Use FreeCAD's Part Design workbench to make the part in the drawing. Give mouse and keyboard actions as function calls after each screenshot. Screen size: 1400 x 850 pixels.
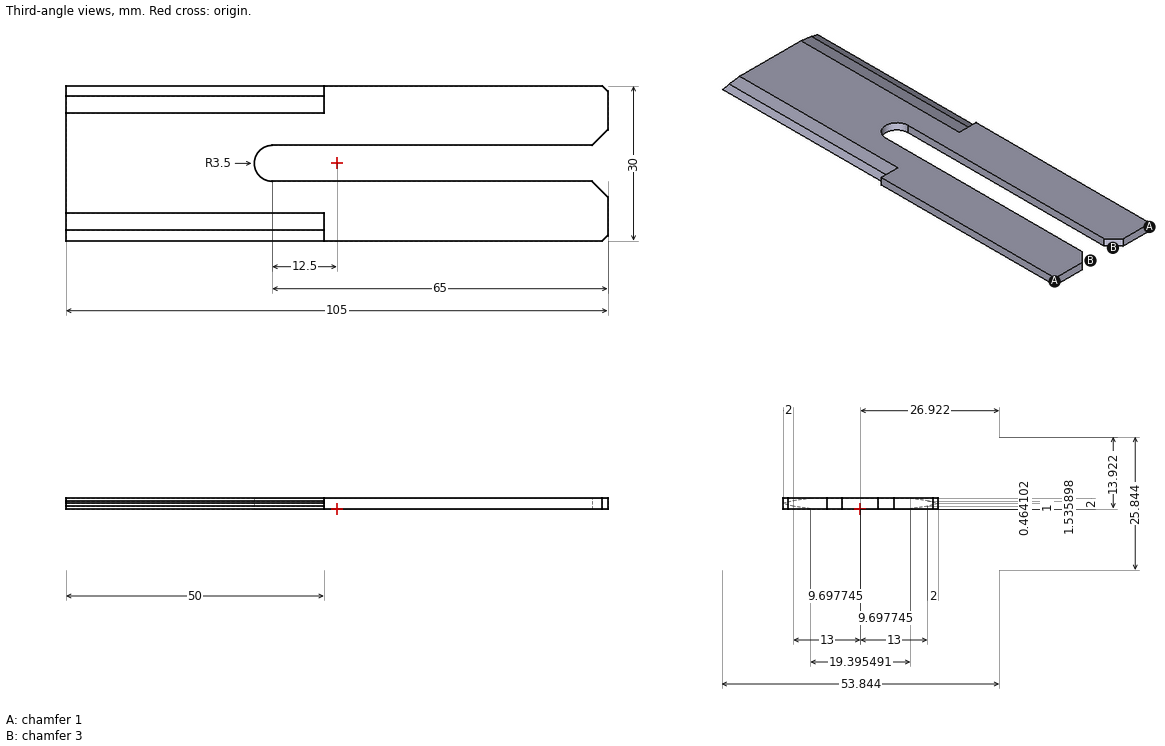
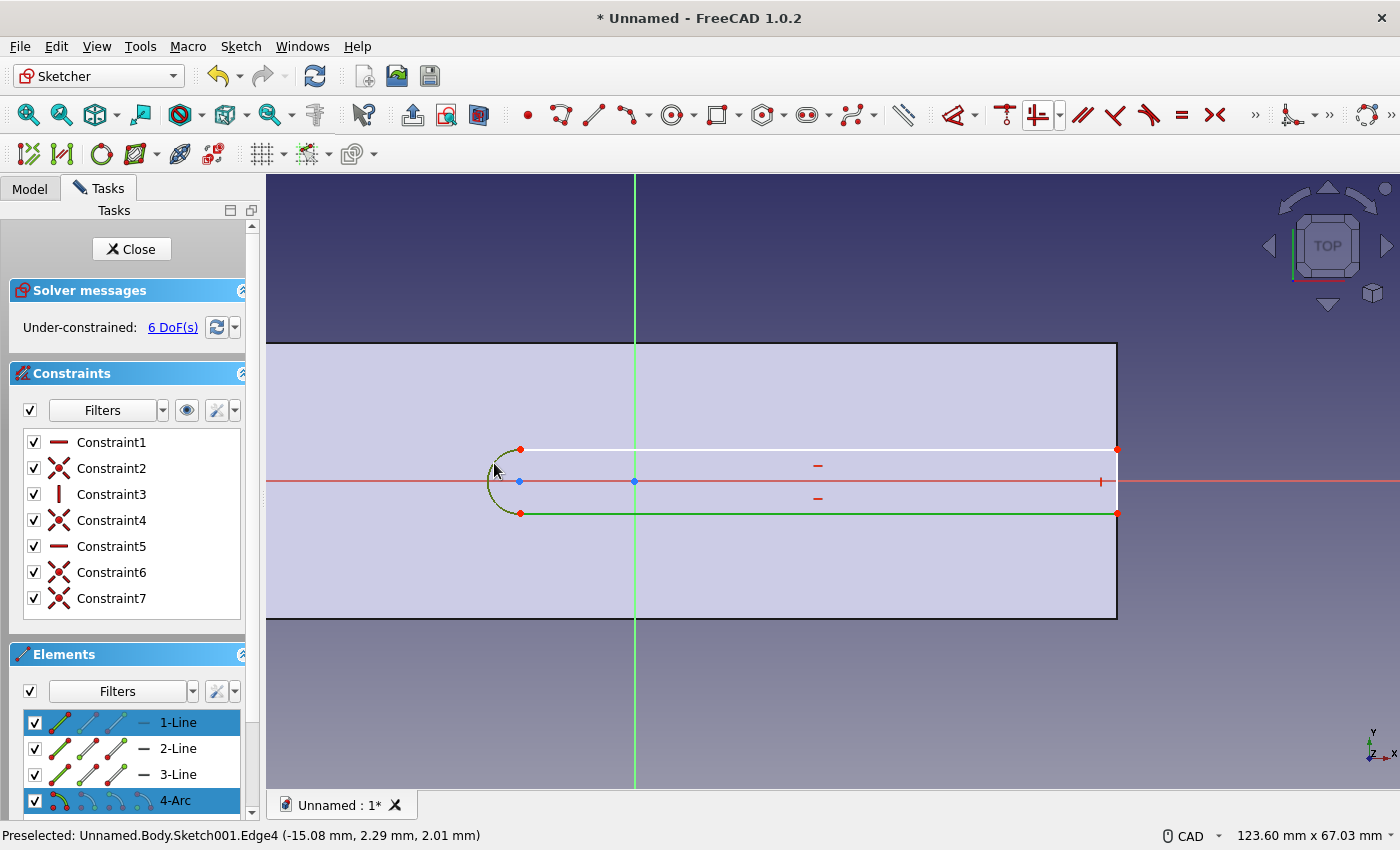
click(1149, 116)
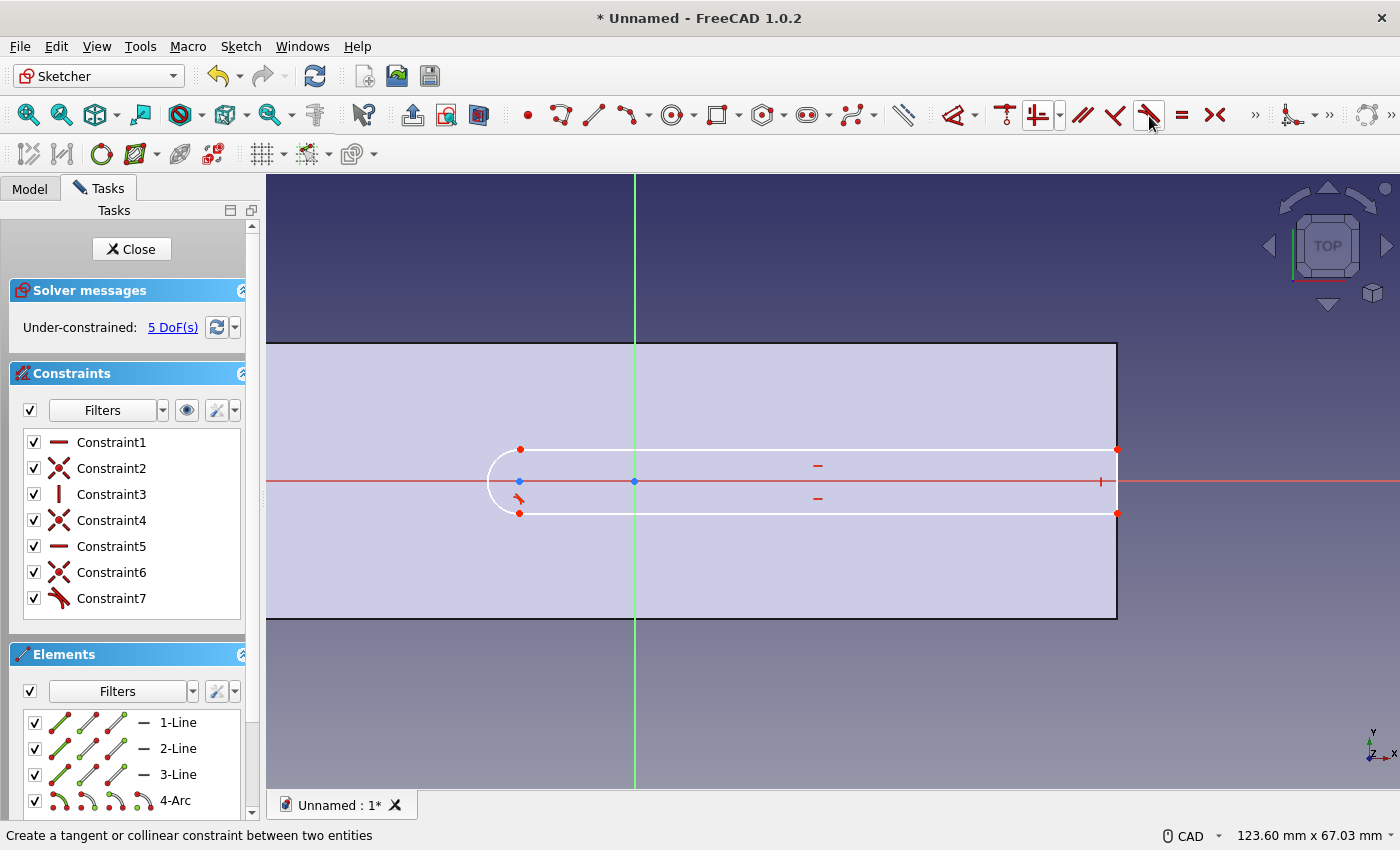
click(938, 450)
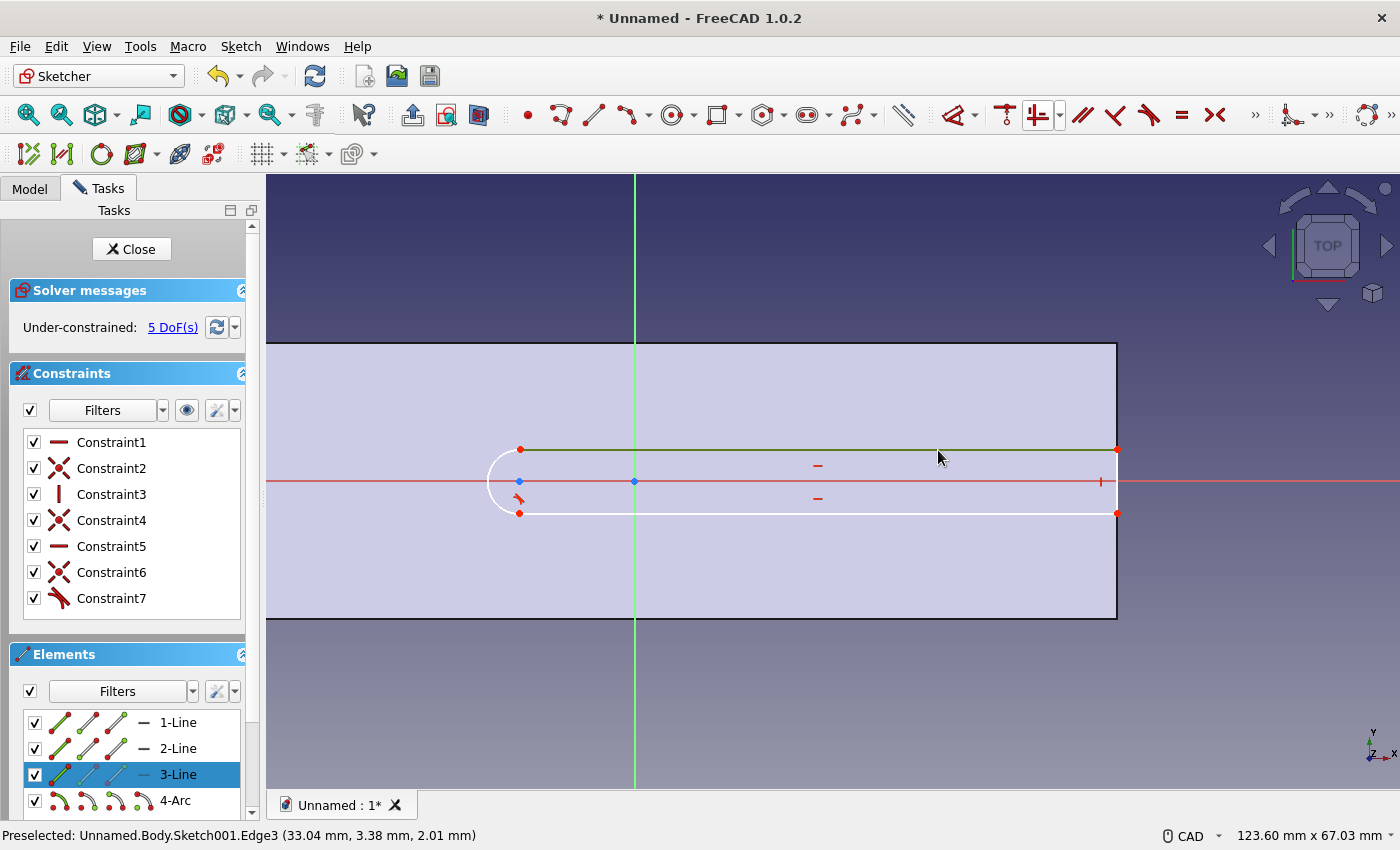
click(494, 463)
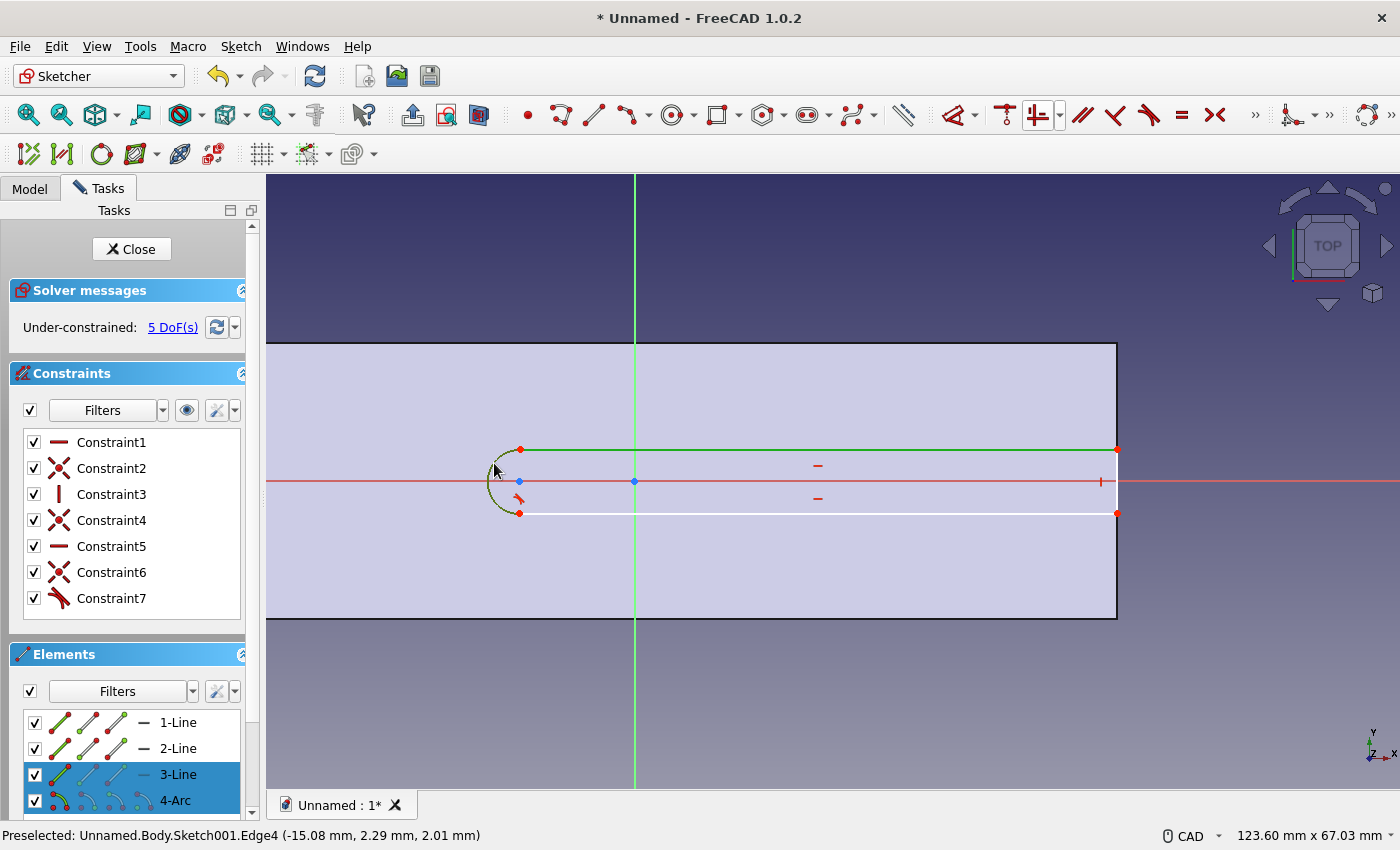
click(1149, 116)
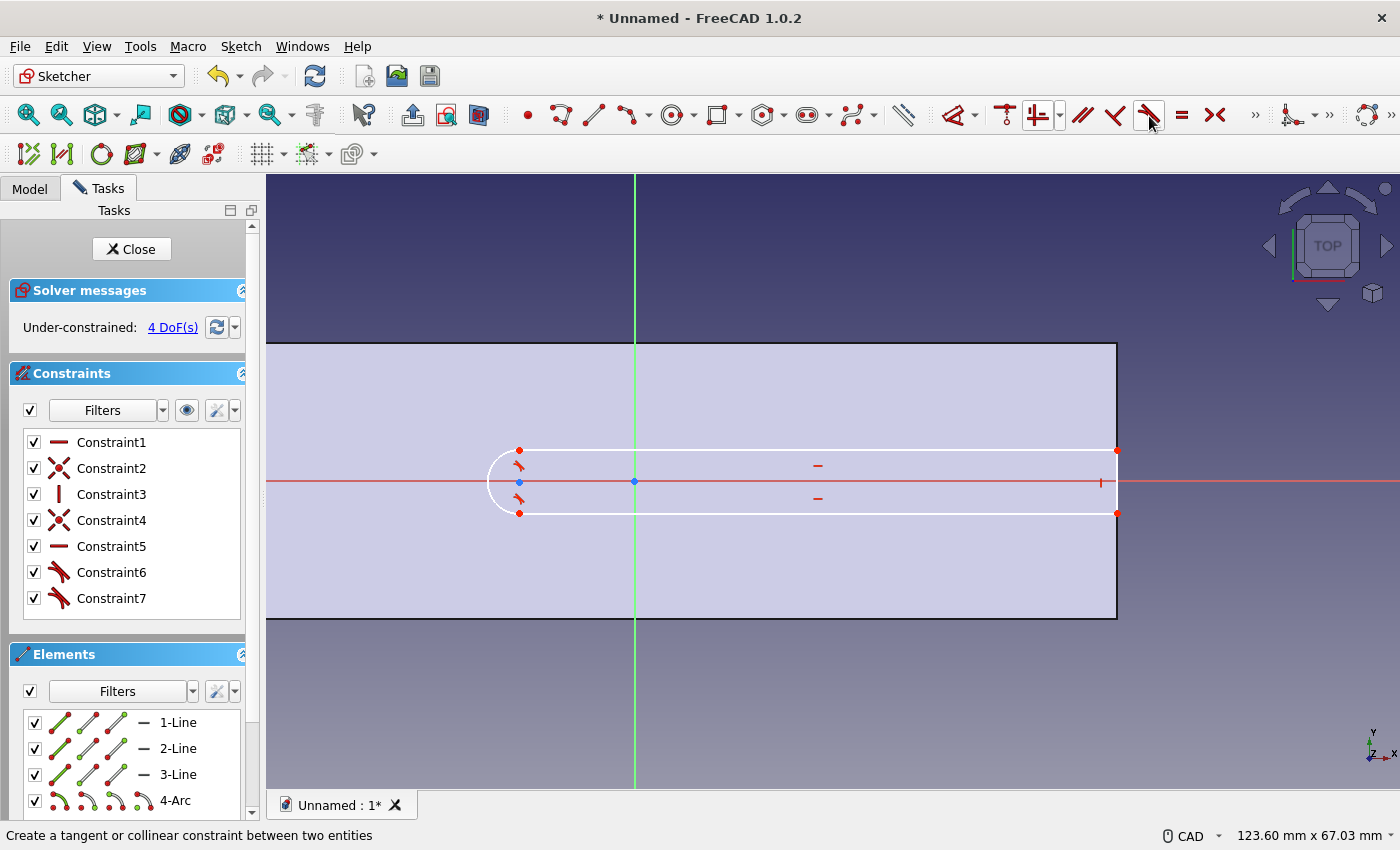
click(520, 482)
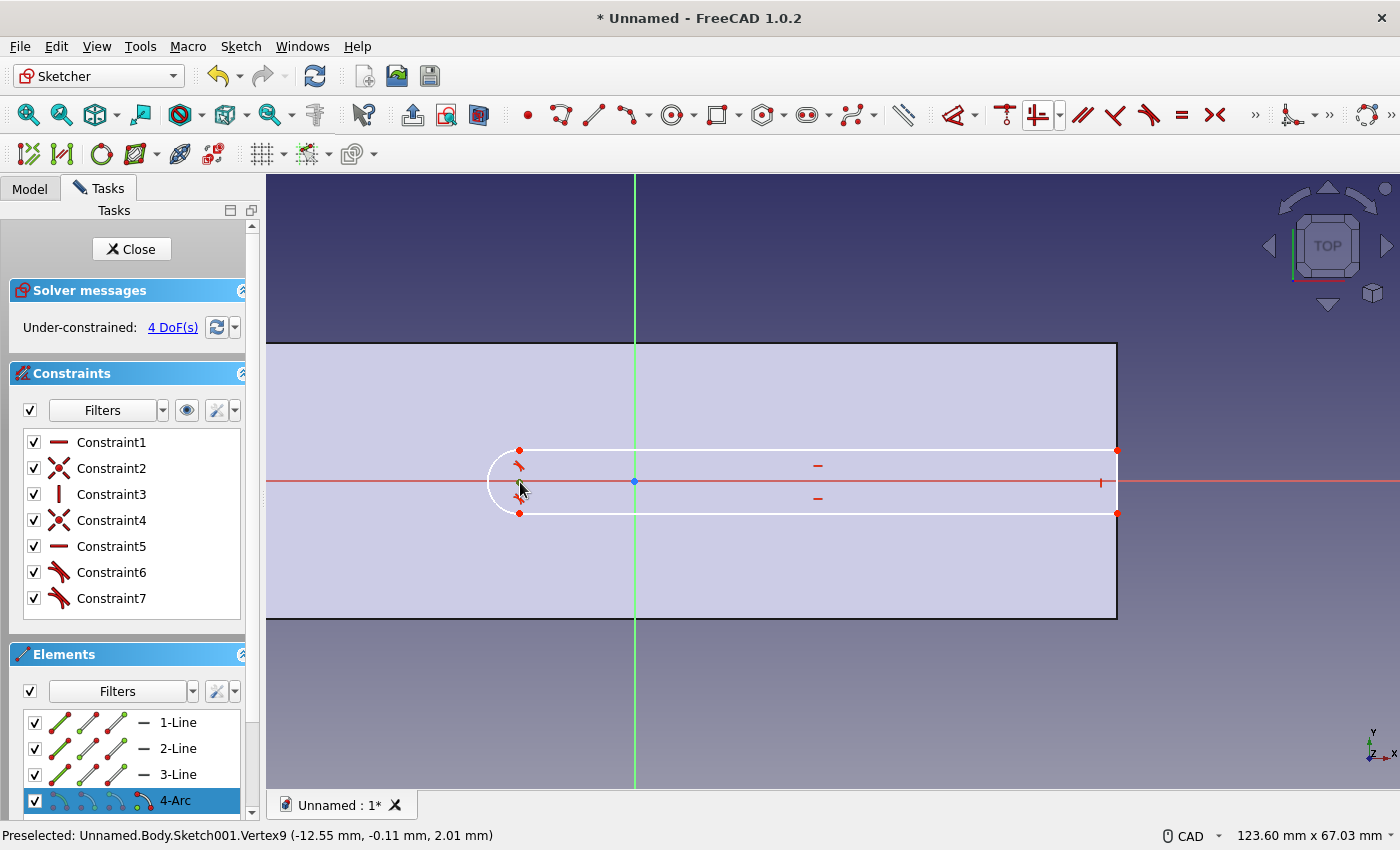
click(361, 481)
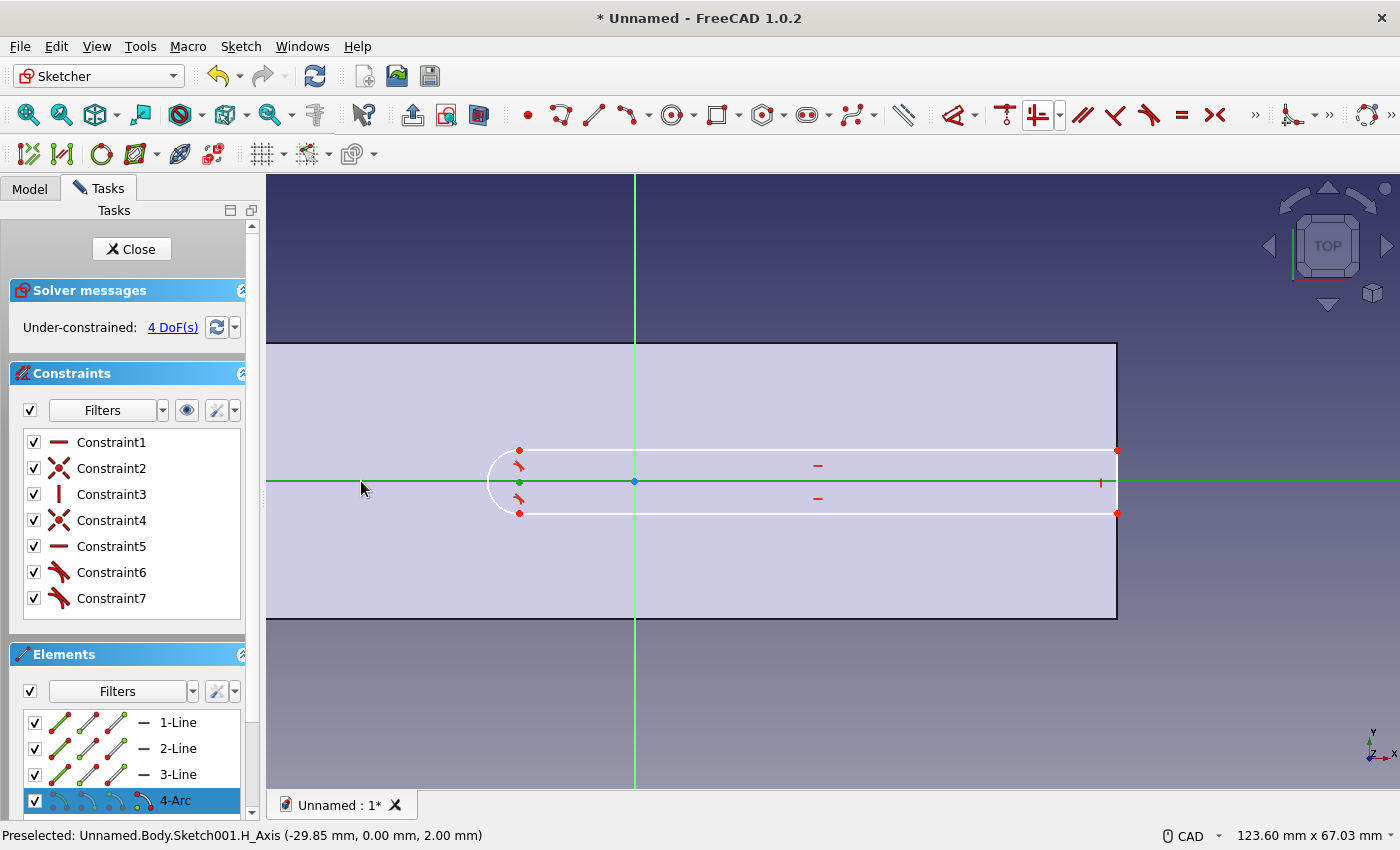
click(1005, 116)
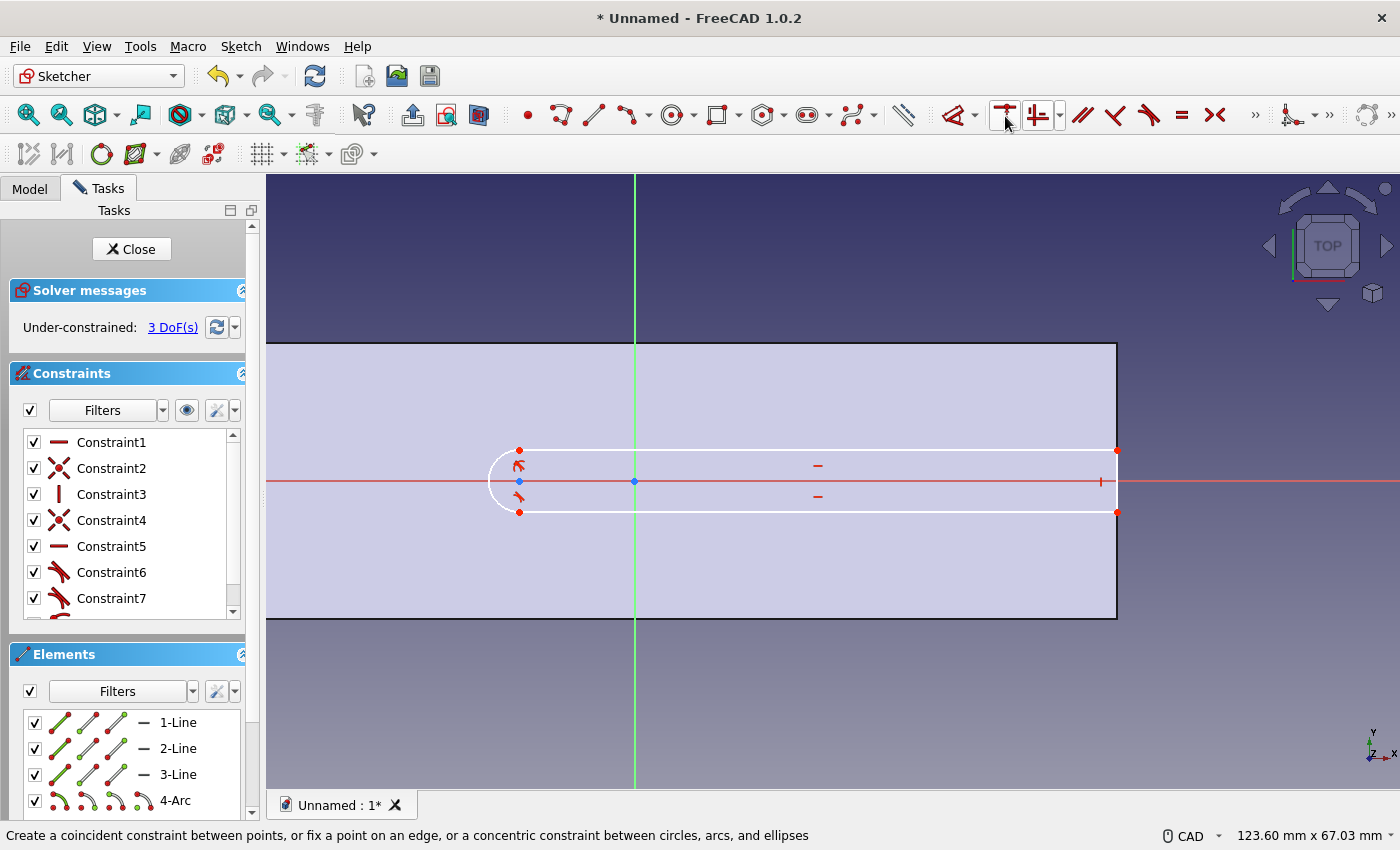
click(952, 116)